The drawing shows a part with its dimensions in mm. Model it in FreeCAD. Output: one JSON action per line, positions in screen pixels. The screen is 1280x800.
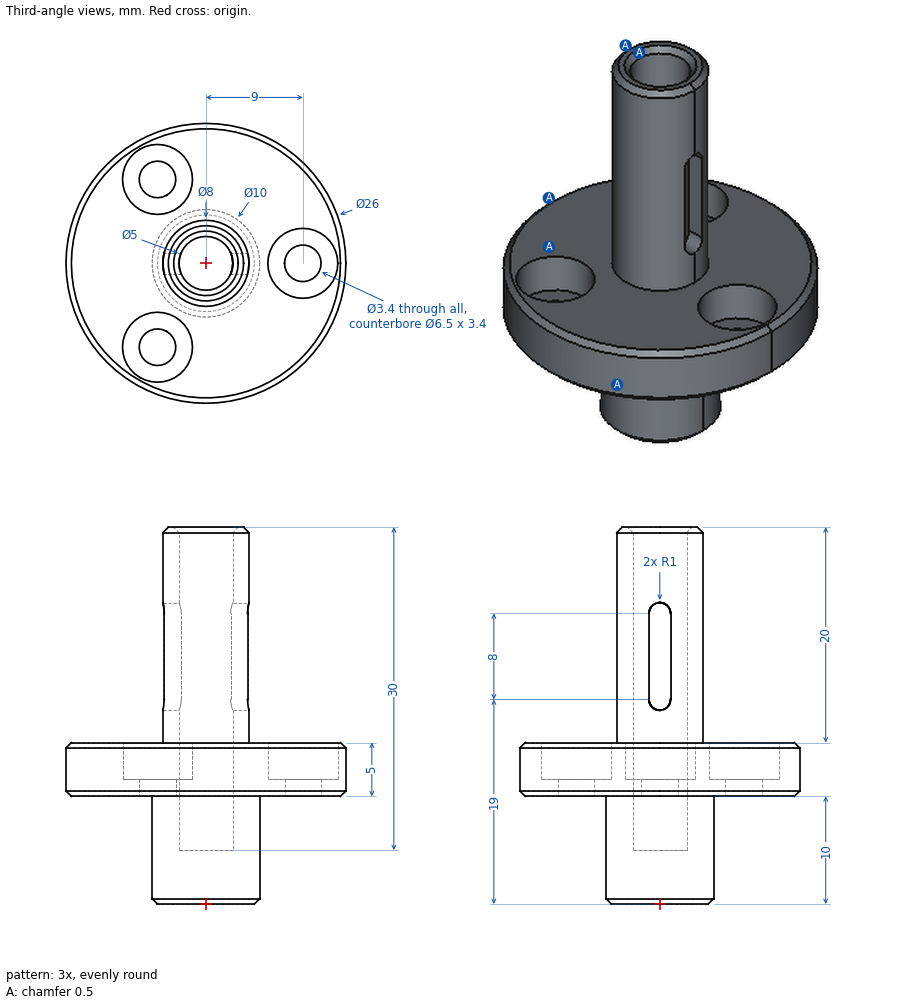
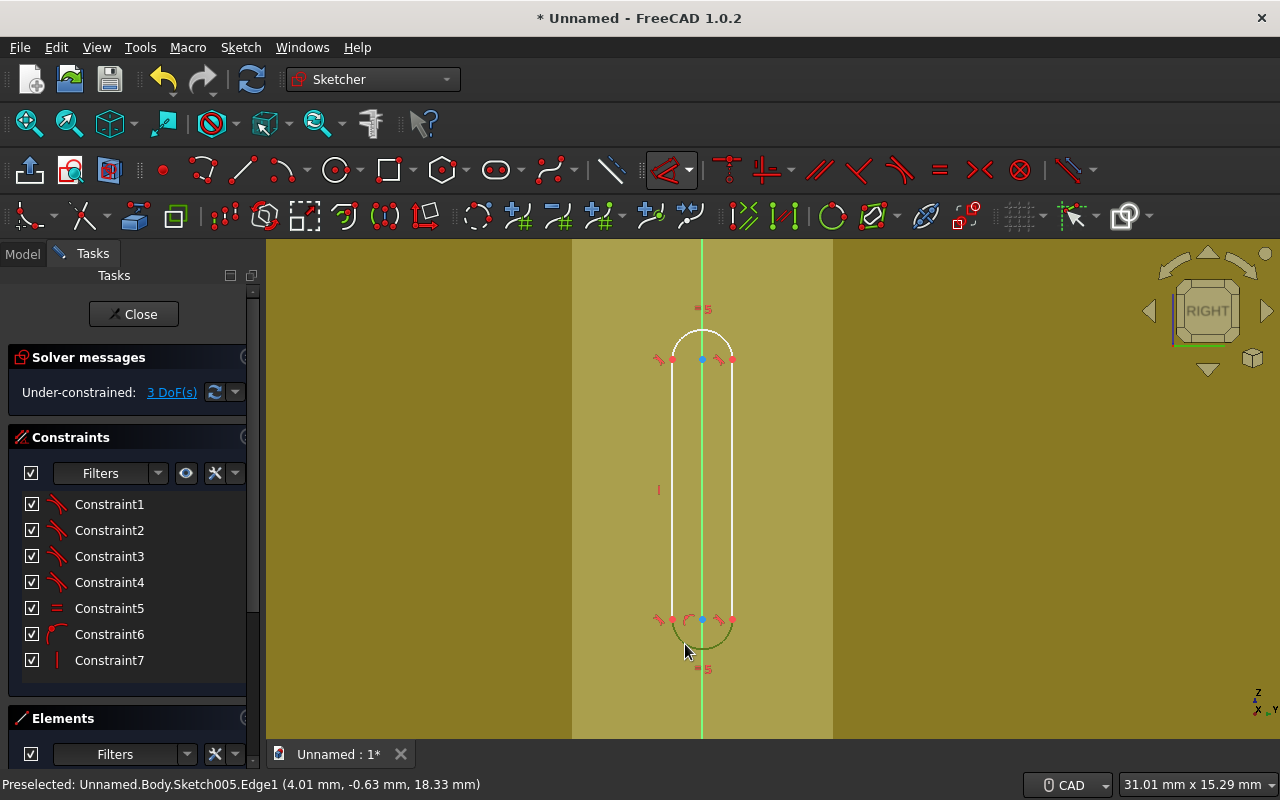
{"action": "left_click", "coordinate": [692, 170]}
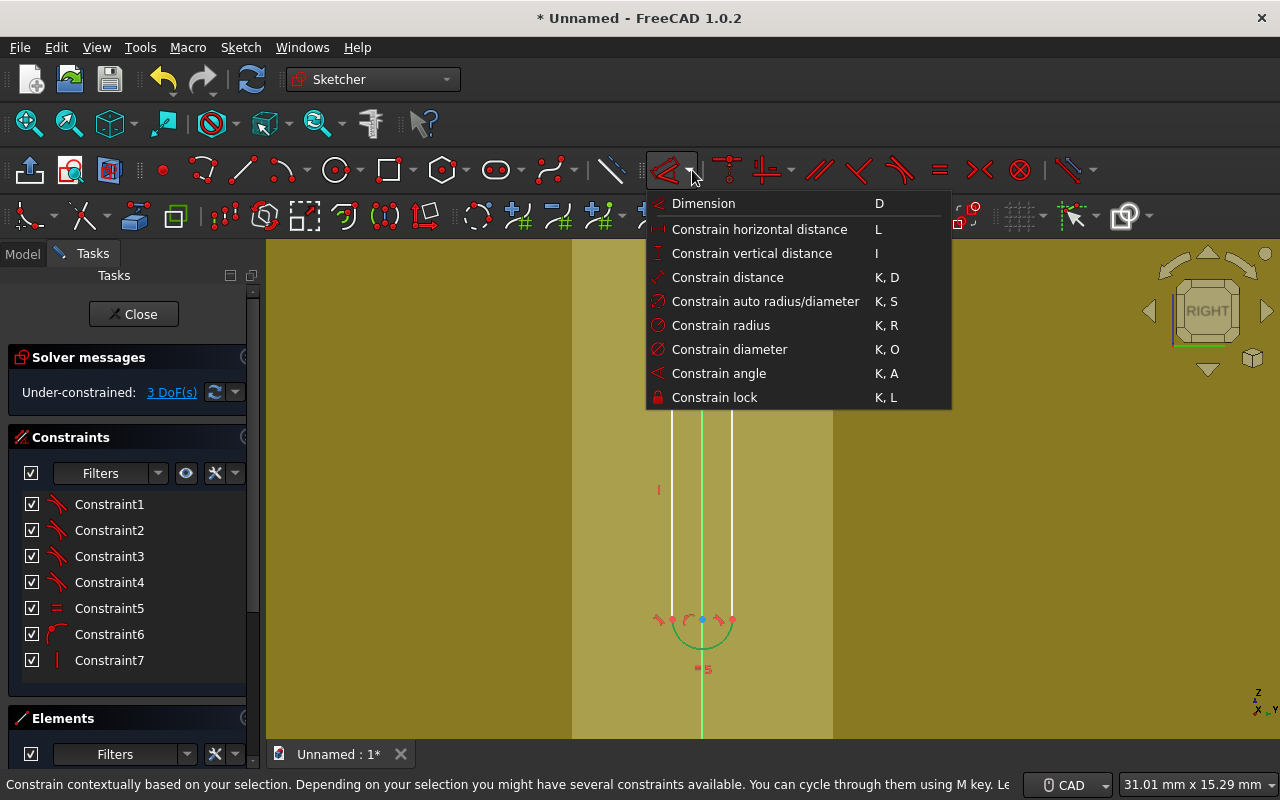
{"action": "left_click", "coordinate": [799, 325]}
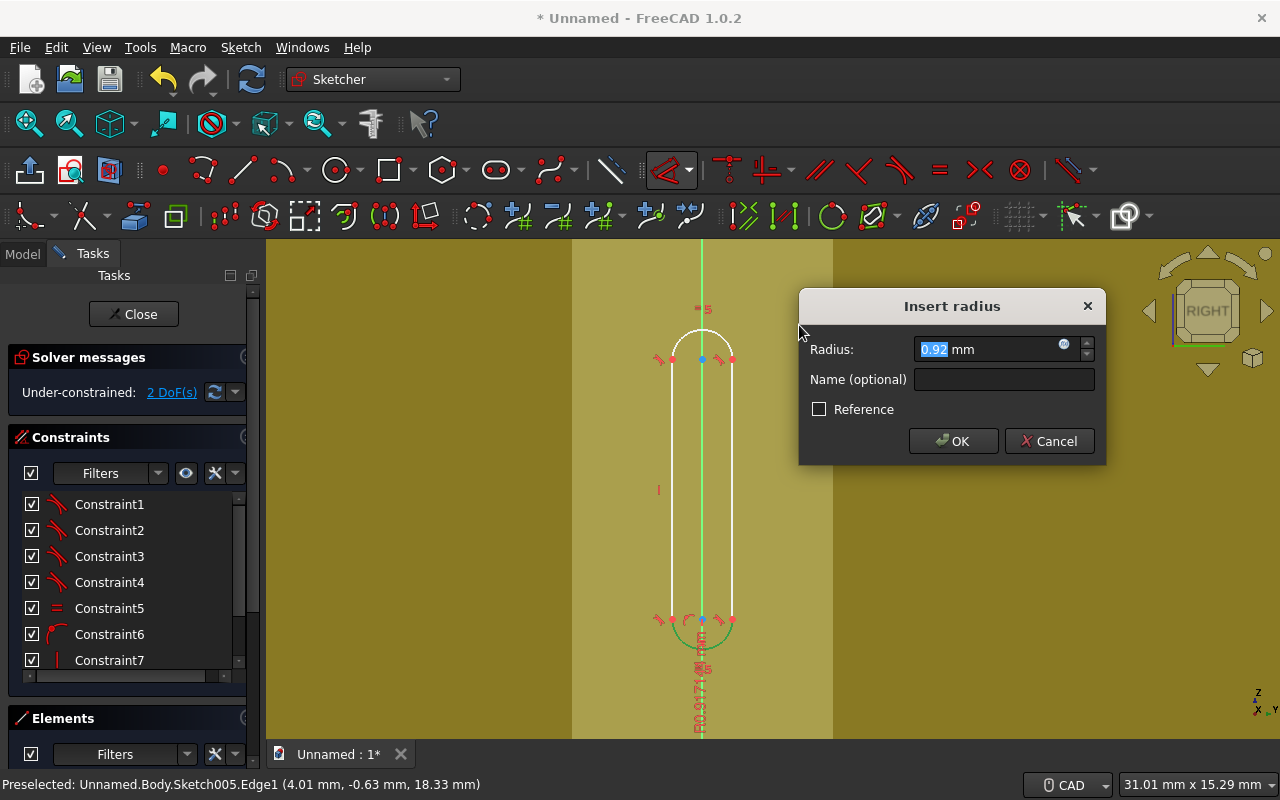
{"action": "type", "text": "1"}
{"action": "key", "text": "Return"}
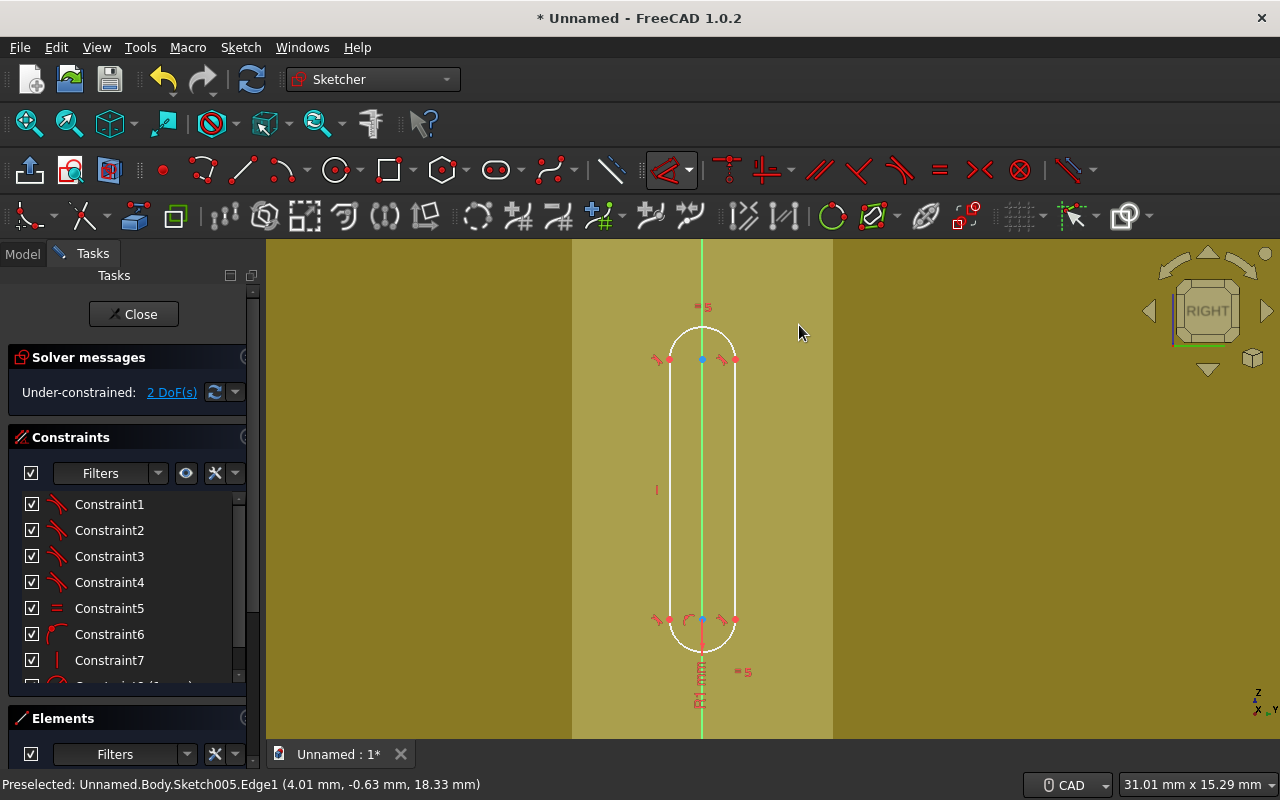
{"action": "left_click", "coordinate": [670, 542]}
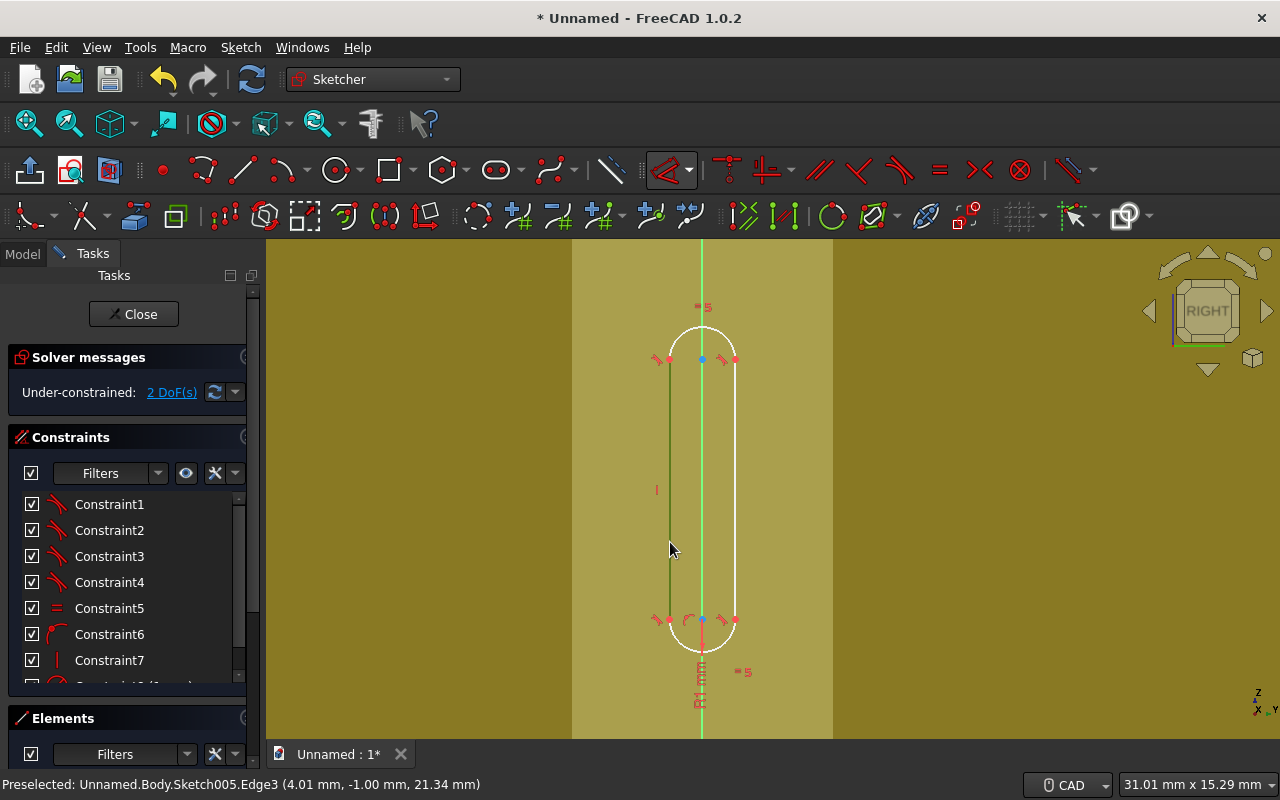
{"action": "left_click", "coordinate": [692, 170]}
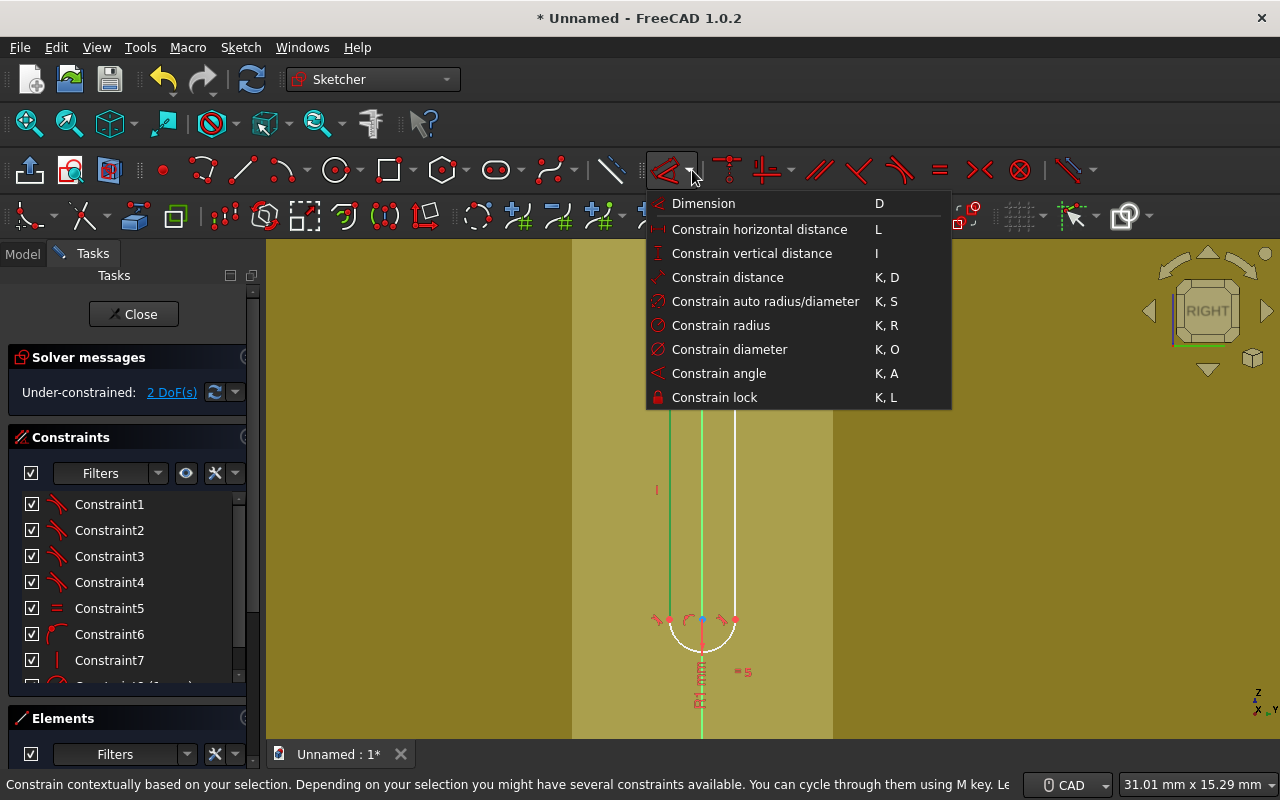
{"action": "left_click", "coordinate": [799, 253]}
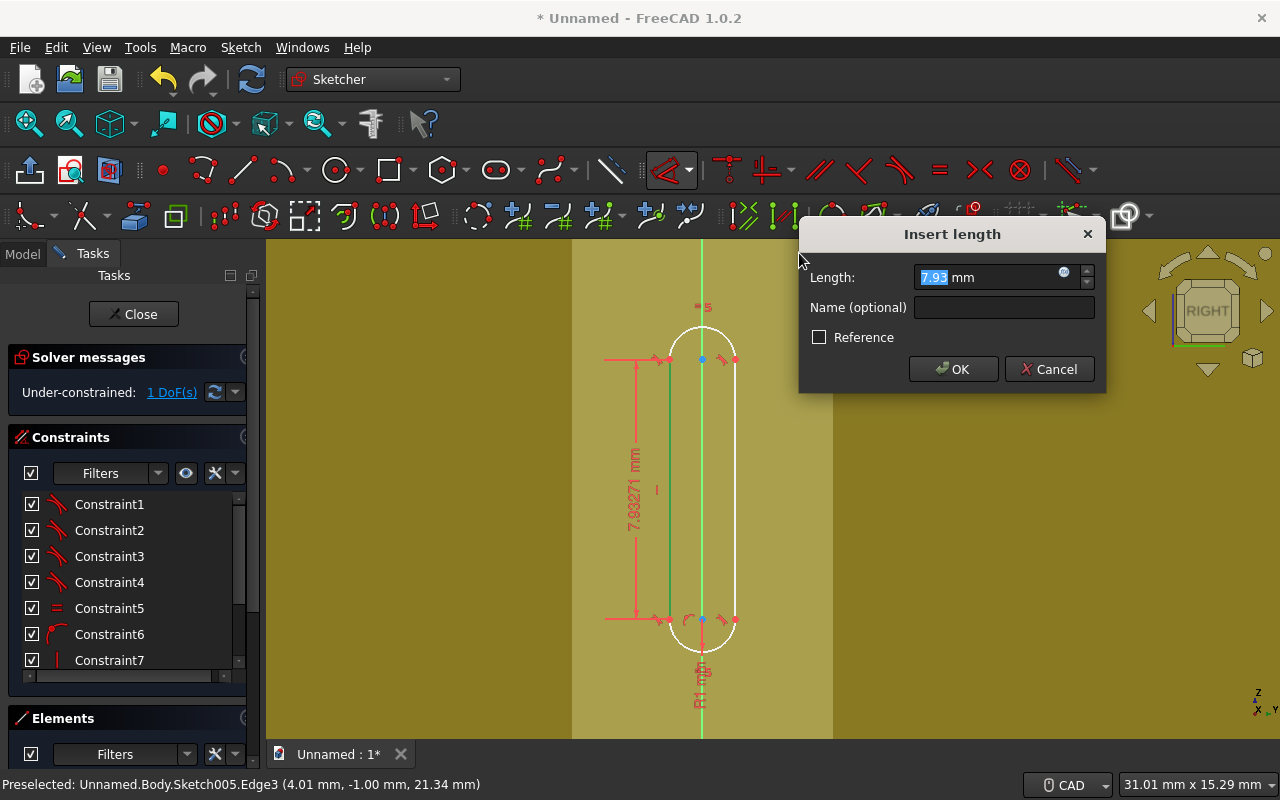
{"action": "type", "text": "8"}
{"action": "key", "text": "Return"}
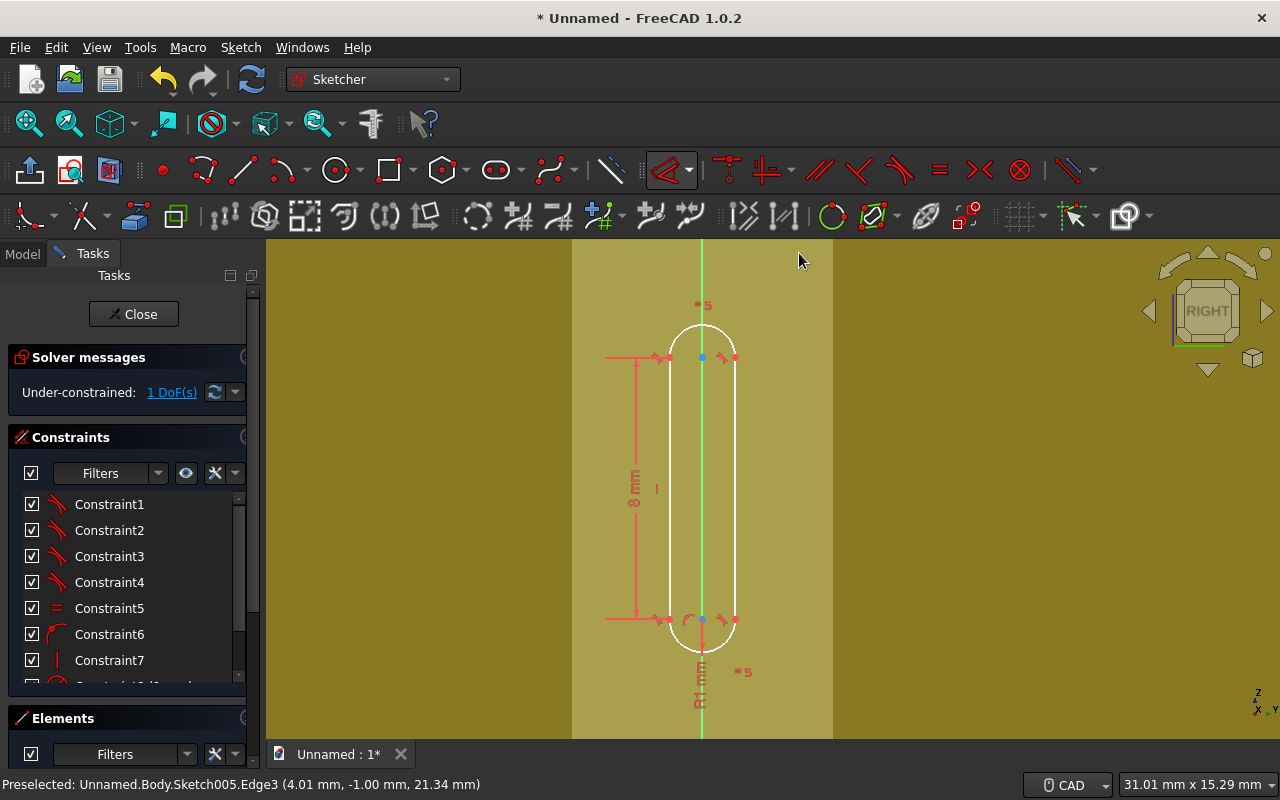
{"action": "left_click", "coordinate": [670, 619]}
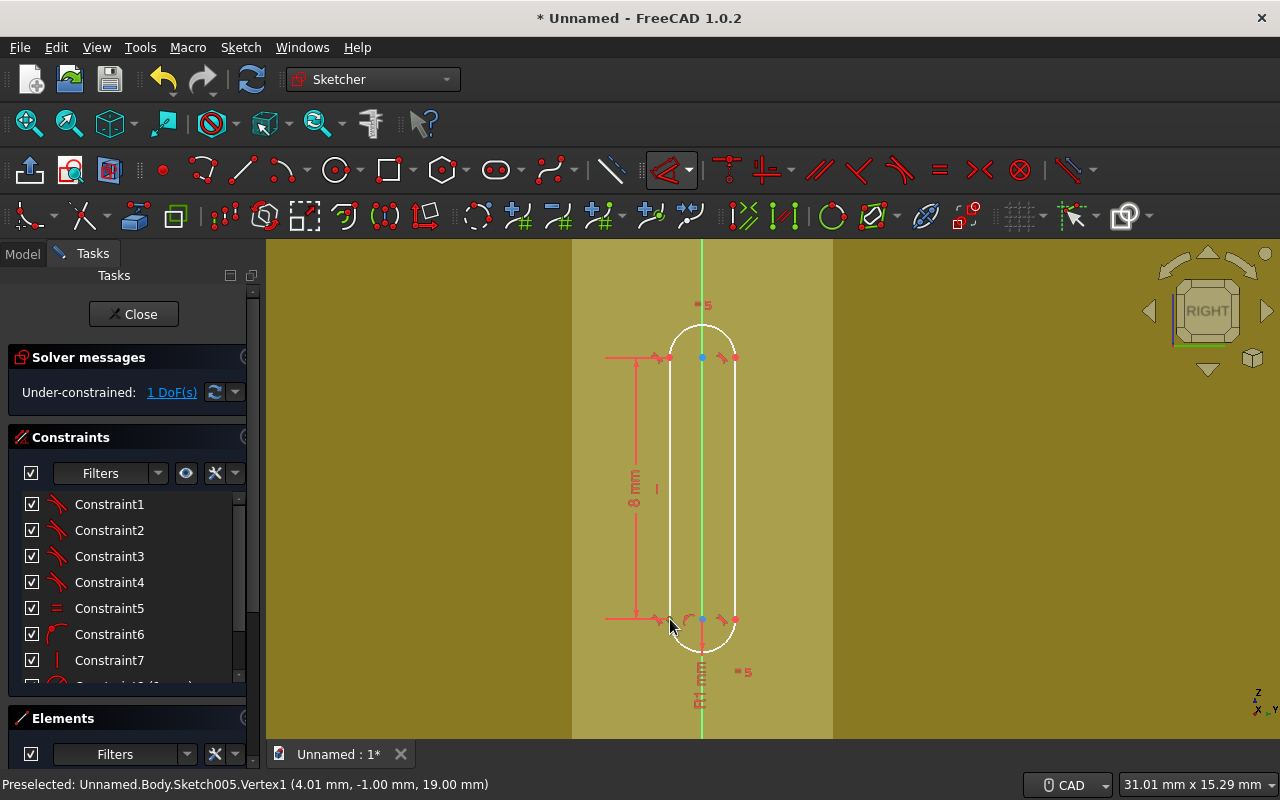
{"action": "left_click", "coordinate": [692, 170]}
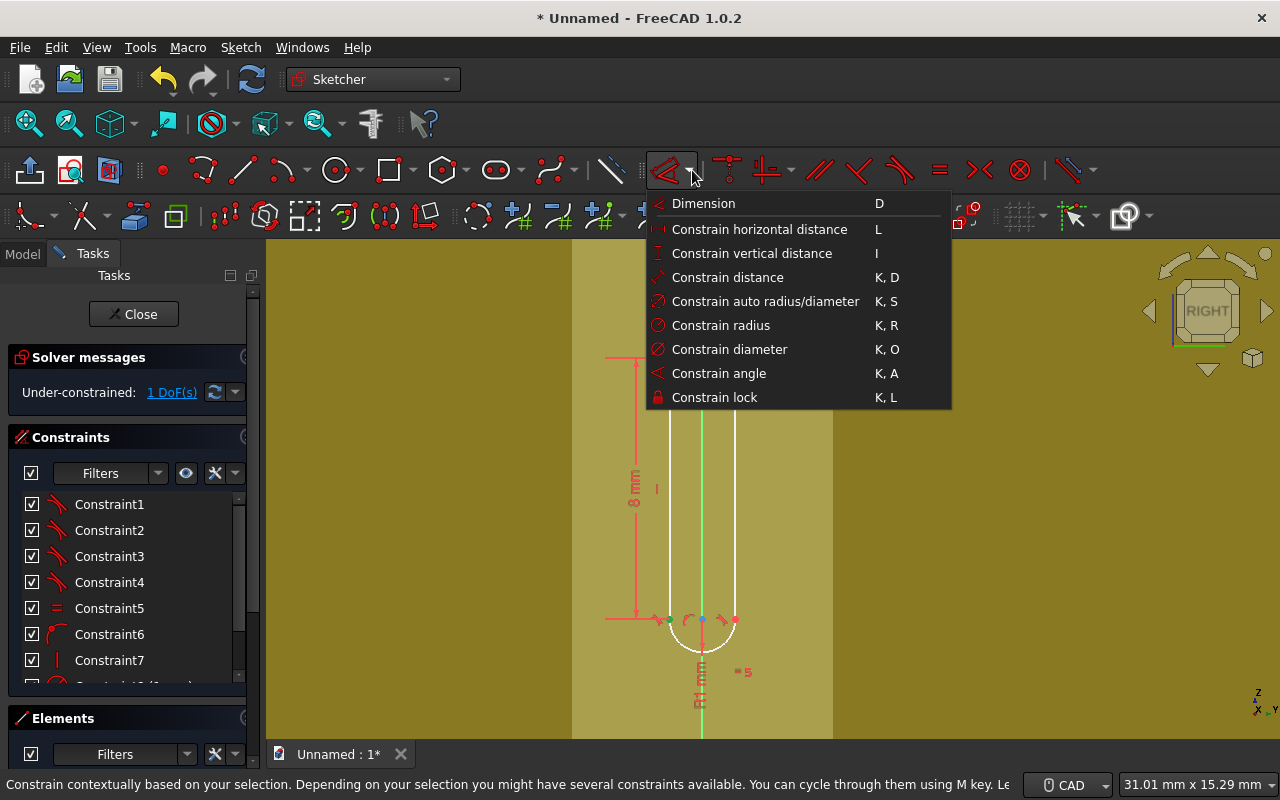
{"action": "left_click", "coordinate": [799, 253]}